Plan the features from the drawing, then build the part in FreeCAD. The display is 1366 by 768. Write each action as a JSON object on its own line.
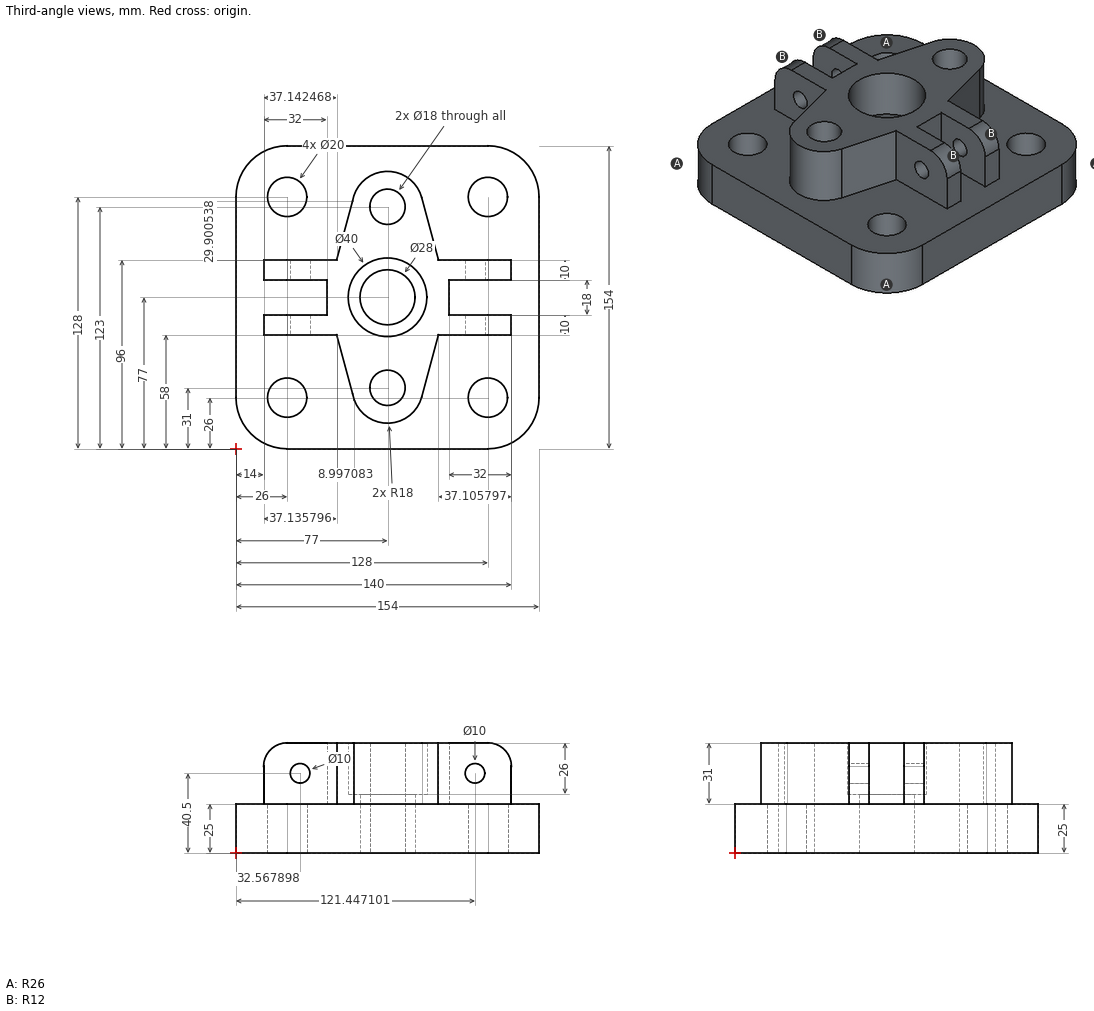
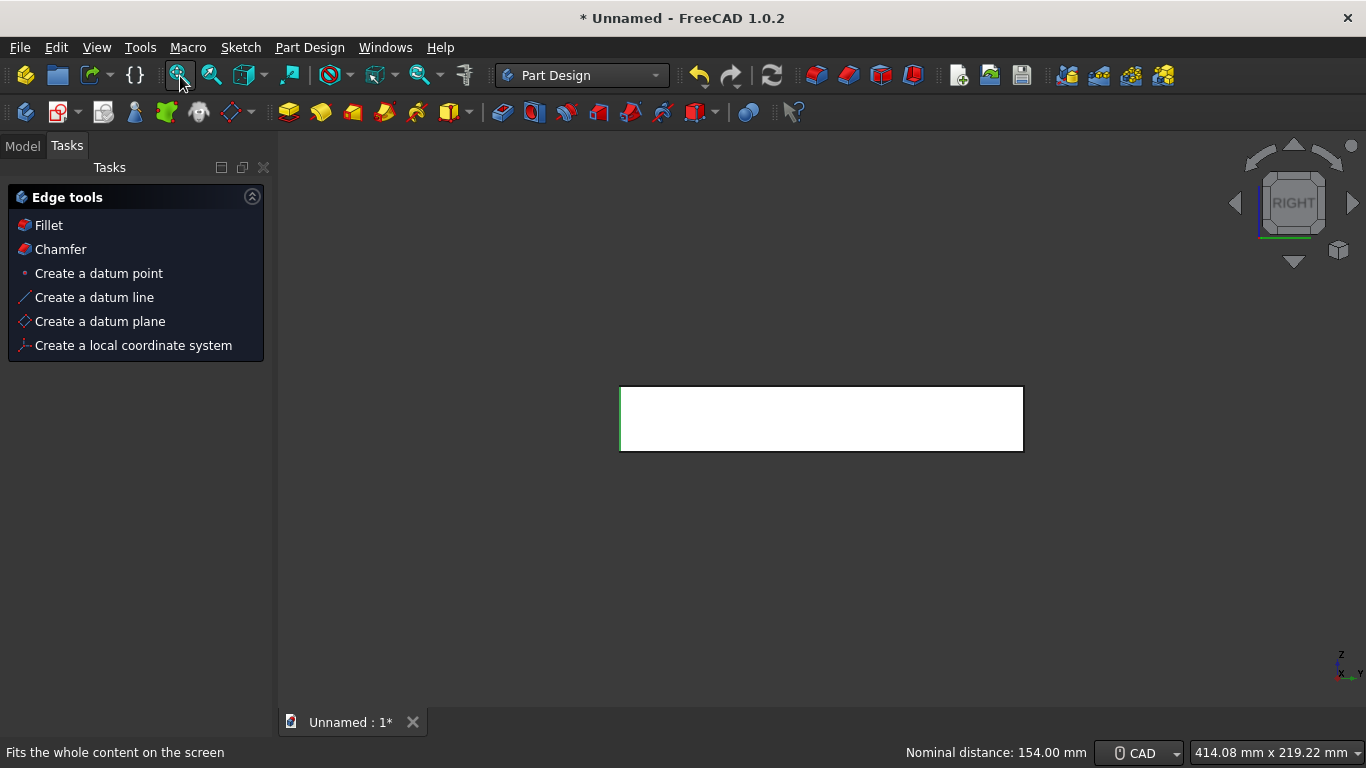
{"action": "left_click", "coordinate": [1024, 418], "text": "ctrl"}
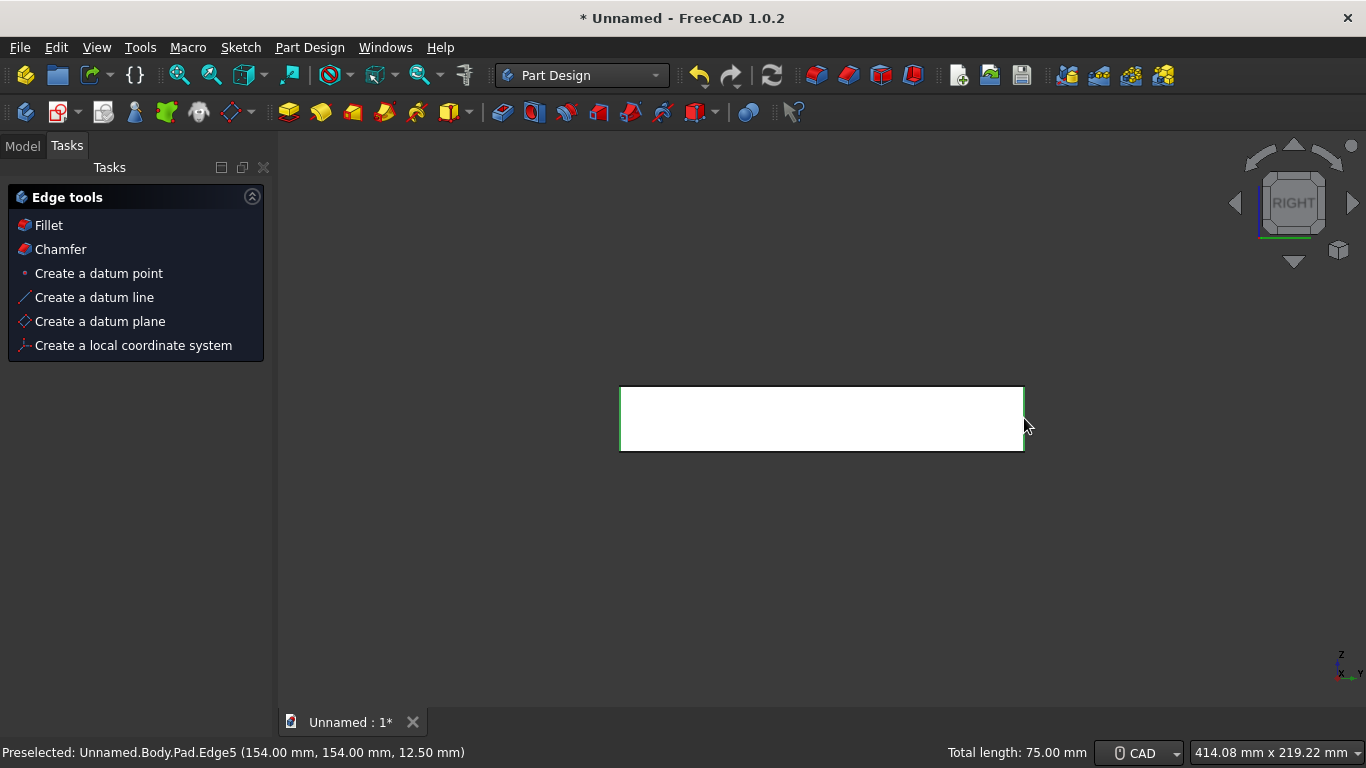
{"action": "key", "text": "5"}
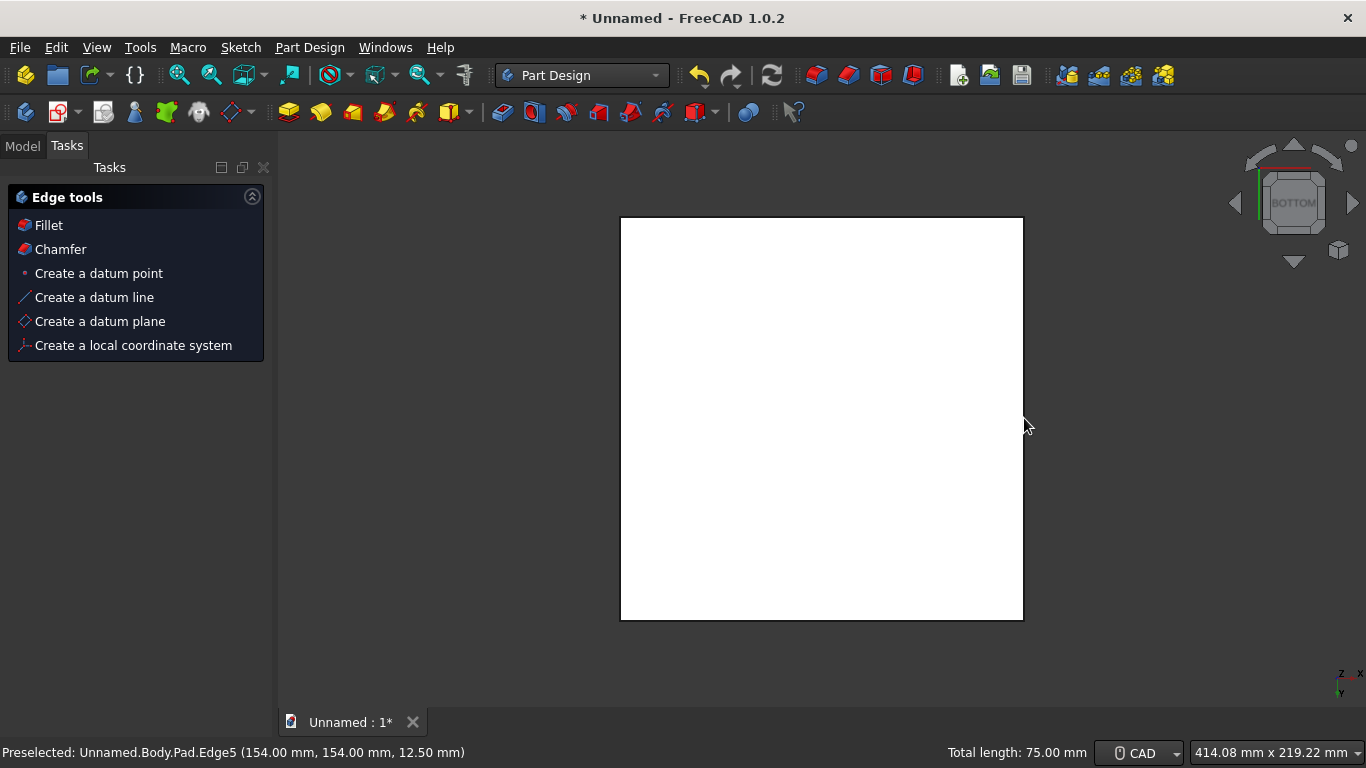
{"action": "key", "text": "4"}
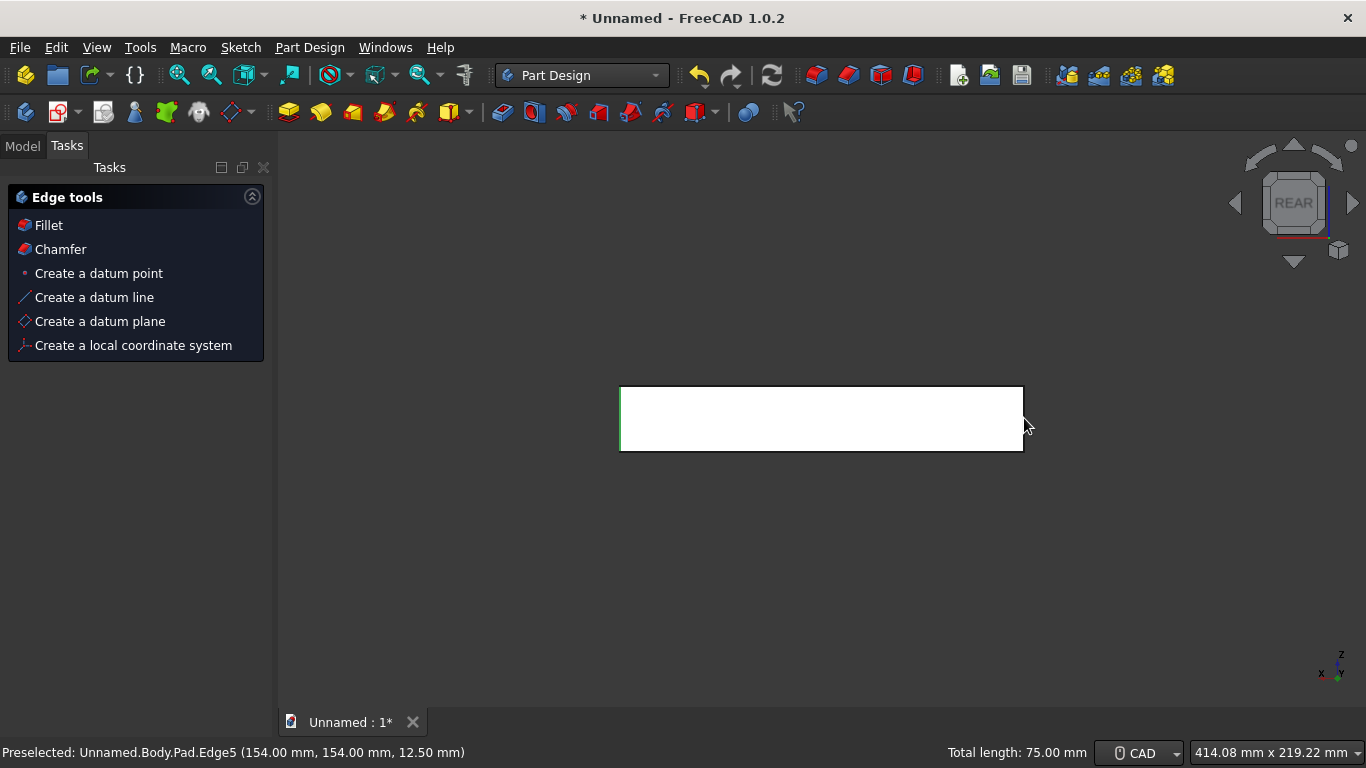
{"action": "left_click", "coordinate": [180, 76]}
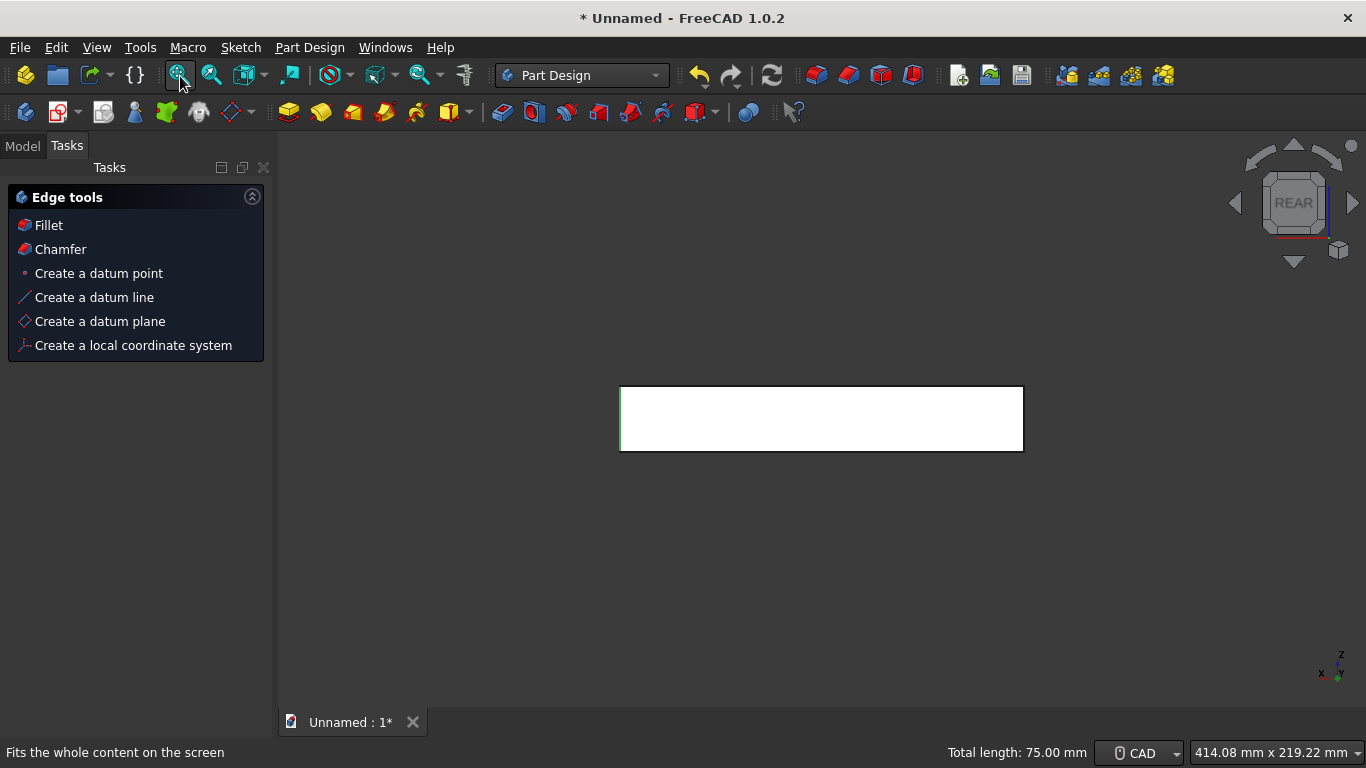
{"action": "left_click", "coordinate": [1024, 418], "text": "ctrl"}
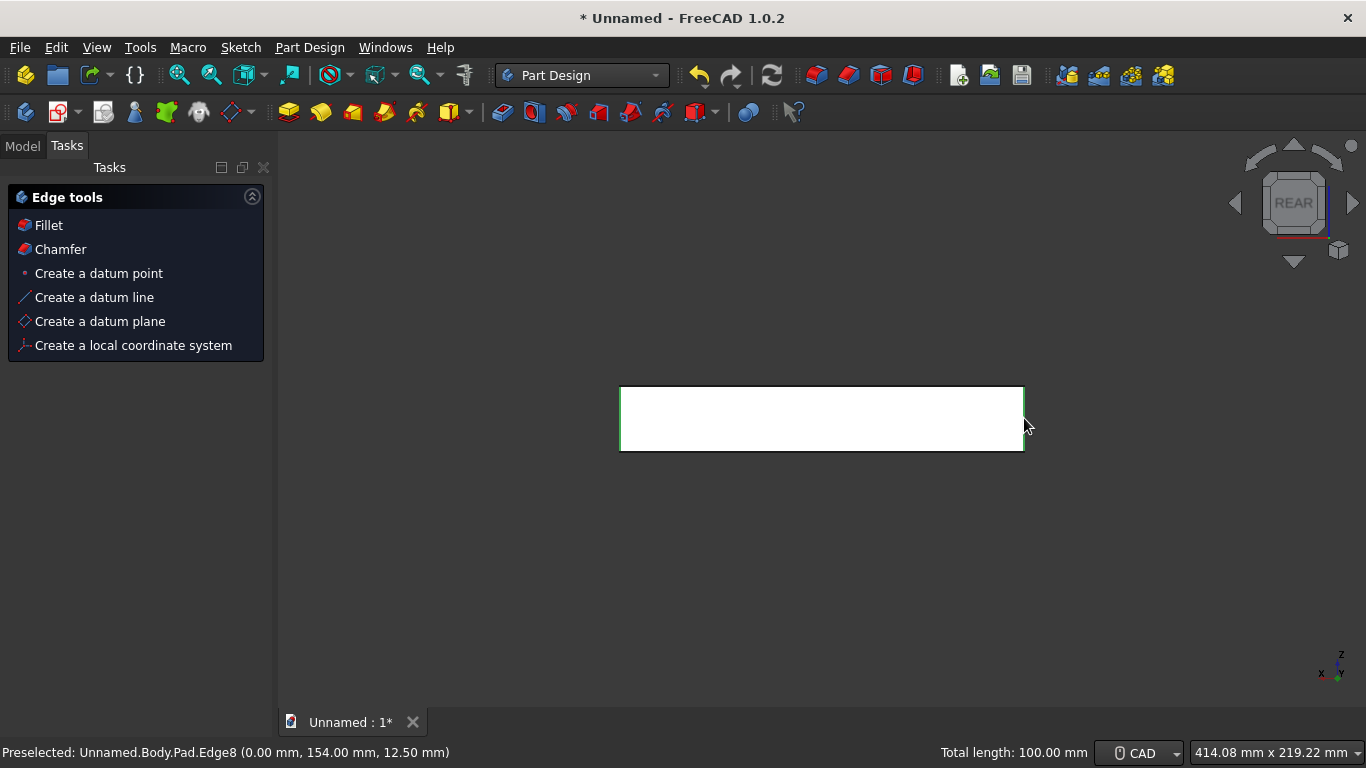
{"action": "left_click", "coordinate": [818, 76]}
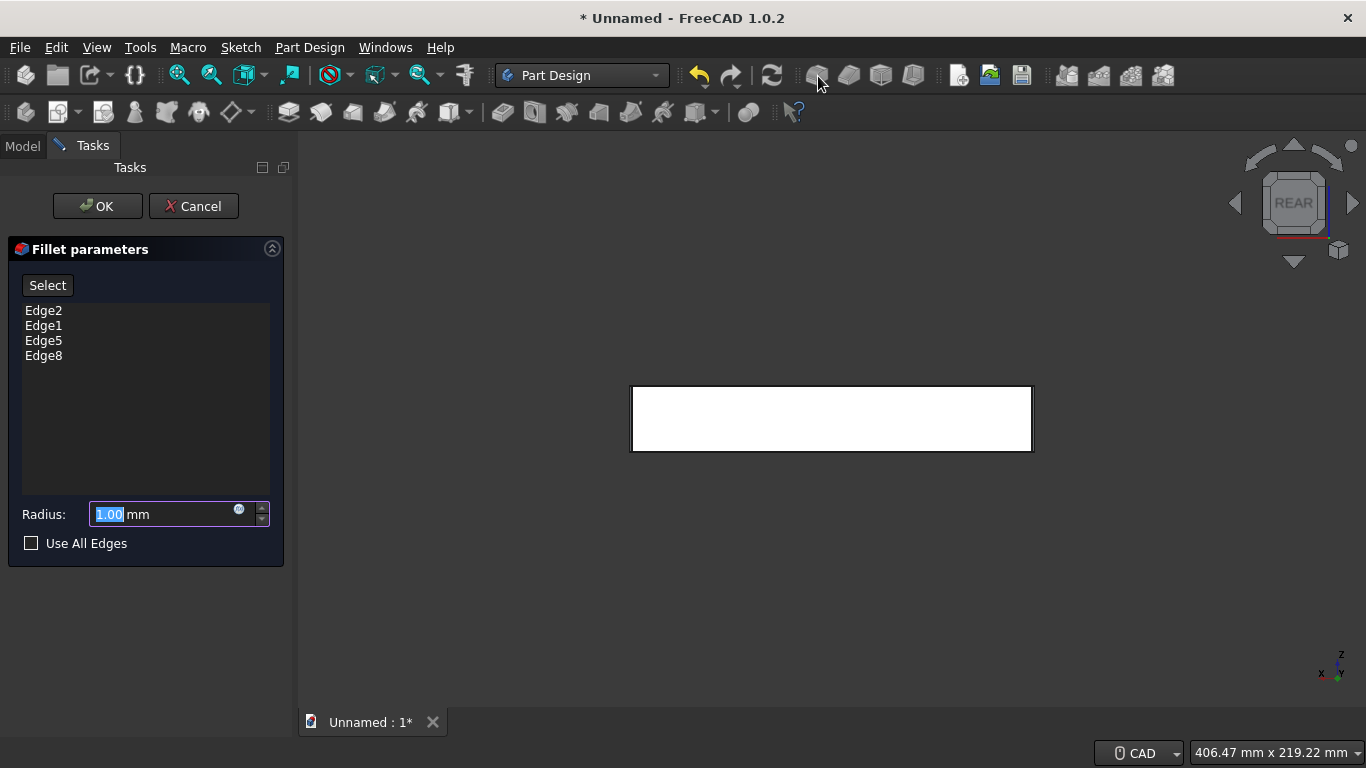
{"action": "type", "text": "26"}
{"action": "key", "text": "Tab"}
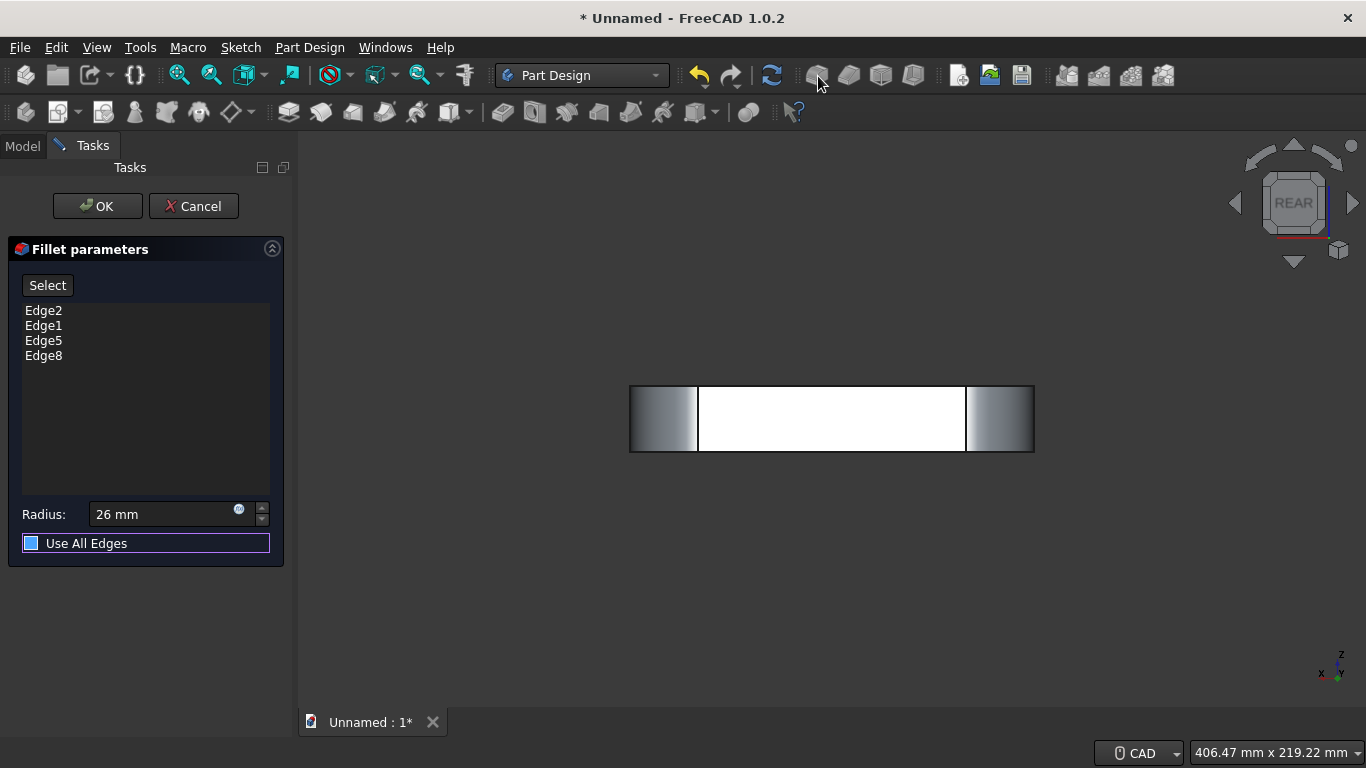
{"action": "left_click", "coordinate": [98, 206]}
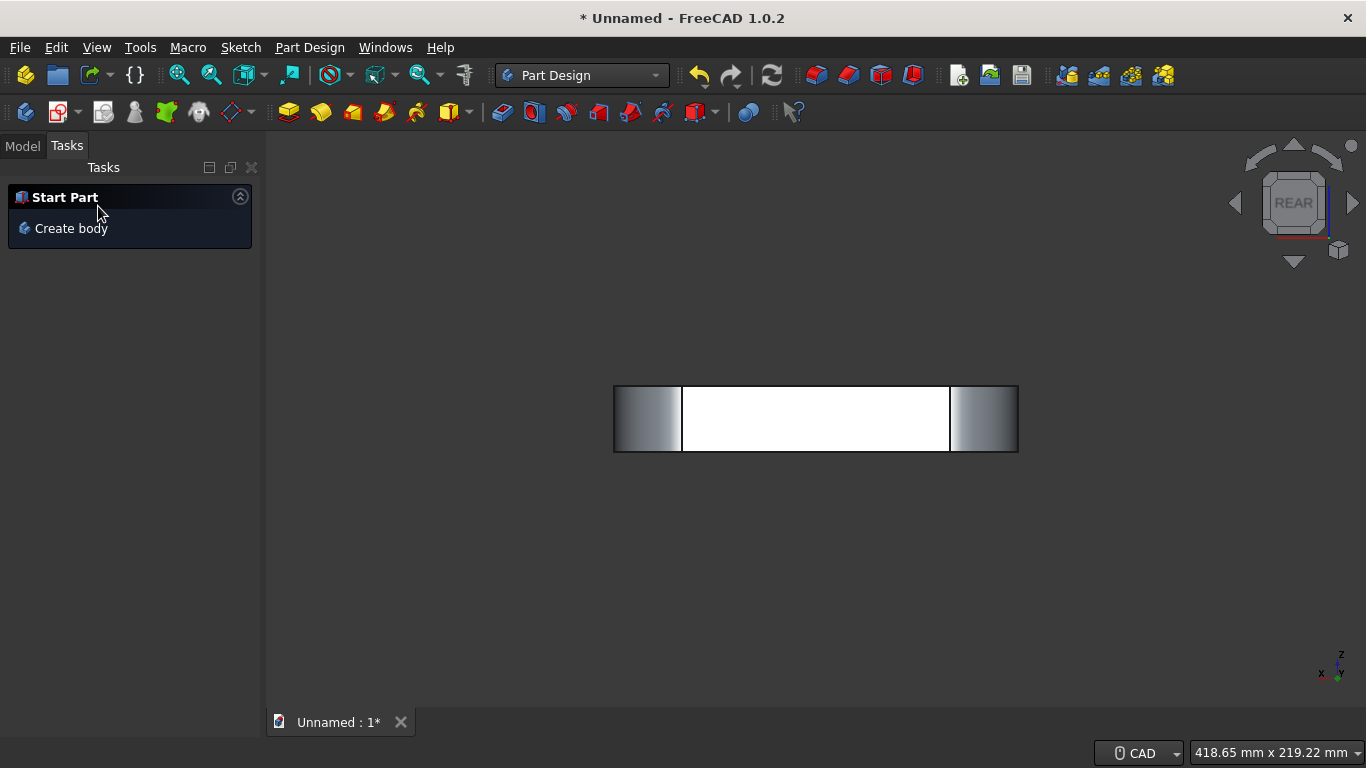
{"action": "left_click", "coordinate": [180, 76]}